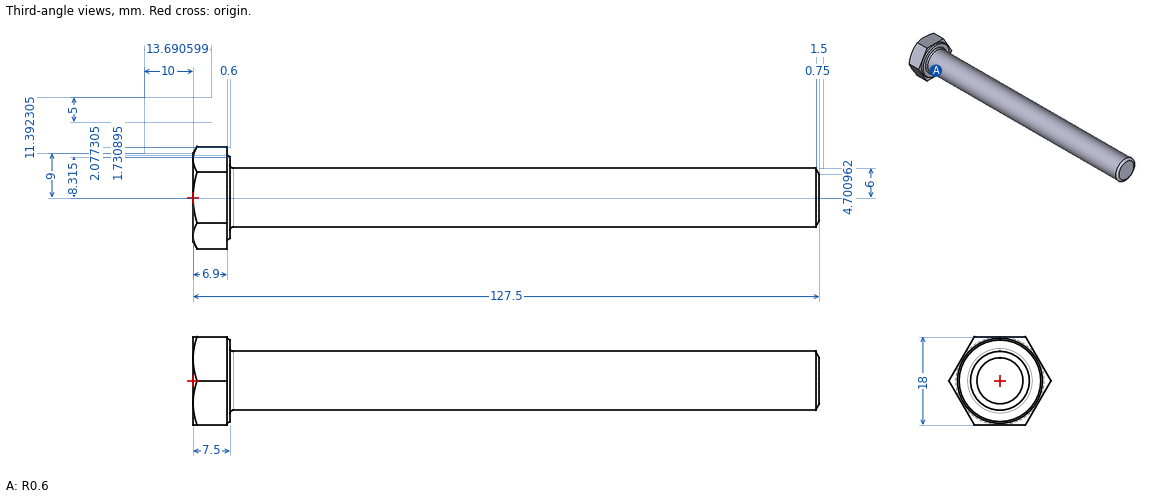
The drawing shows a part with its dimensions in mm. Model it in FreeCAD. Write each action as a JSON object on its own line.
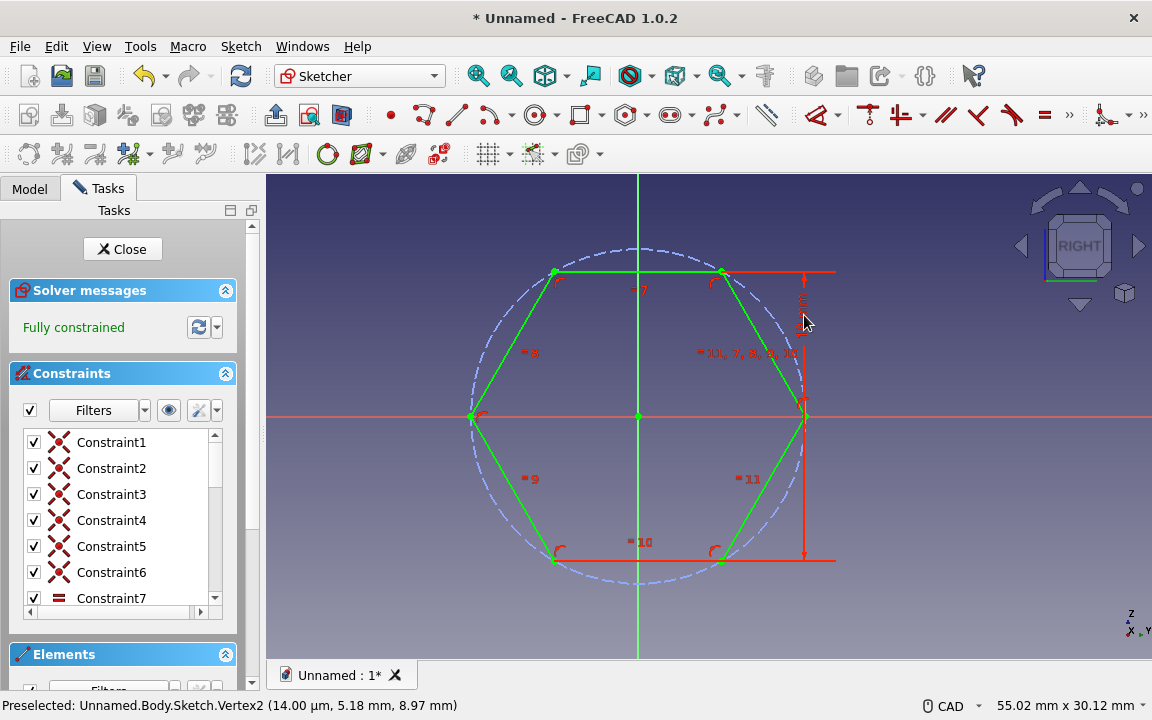
{"action": "left_click", "coordinate": [123, 249]}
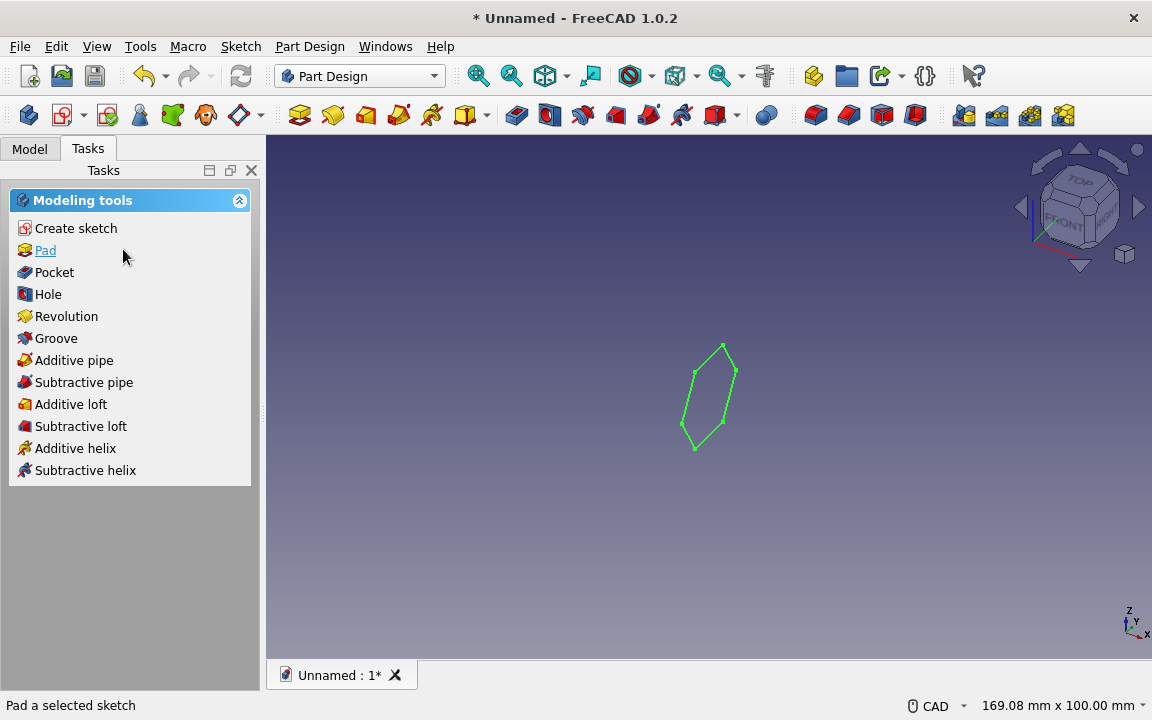
{"action": "left_click", "coordinate": [300, 116]}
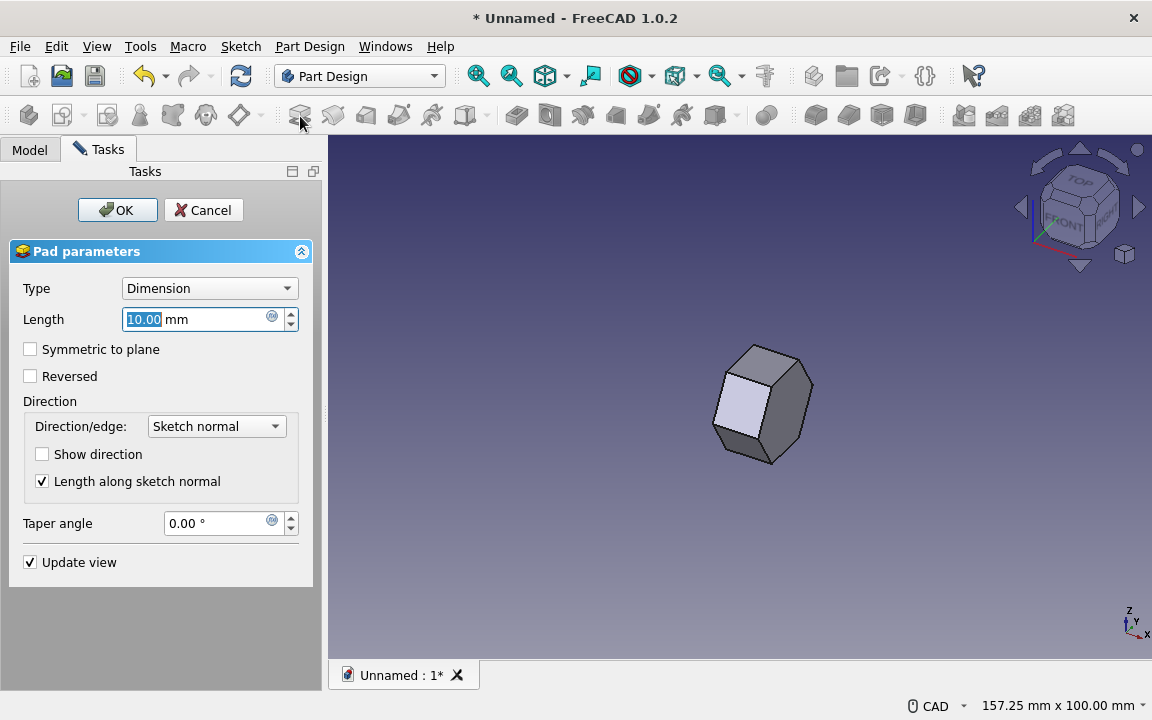
{"action": "type", "text": "7.5"}
{"action": "key", "text": "Tab"}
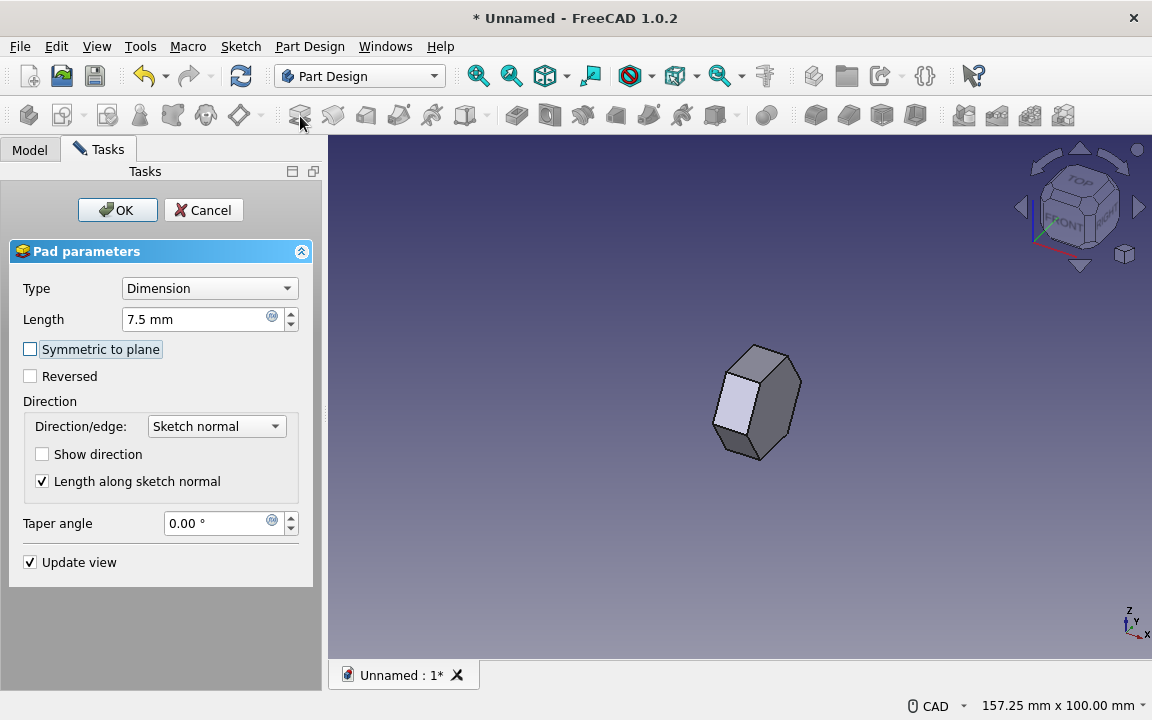
{"action": "left_click", "coordinate": [118, 210]}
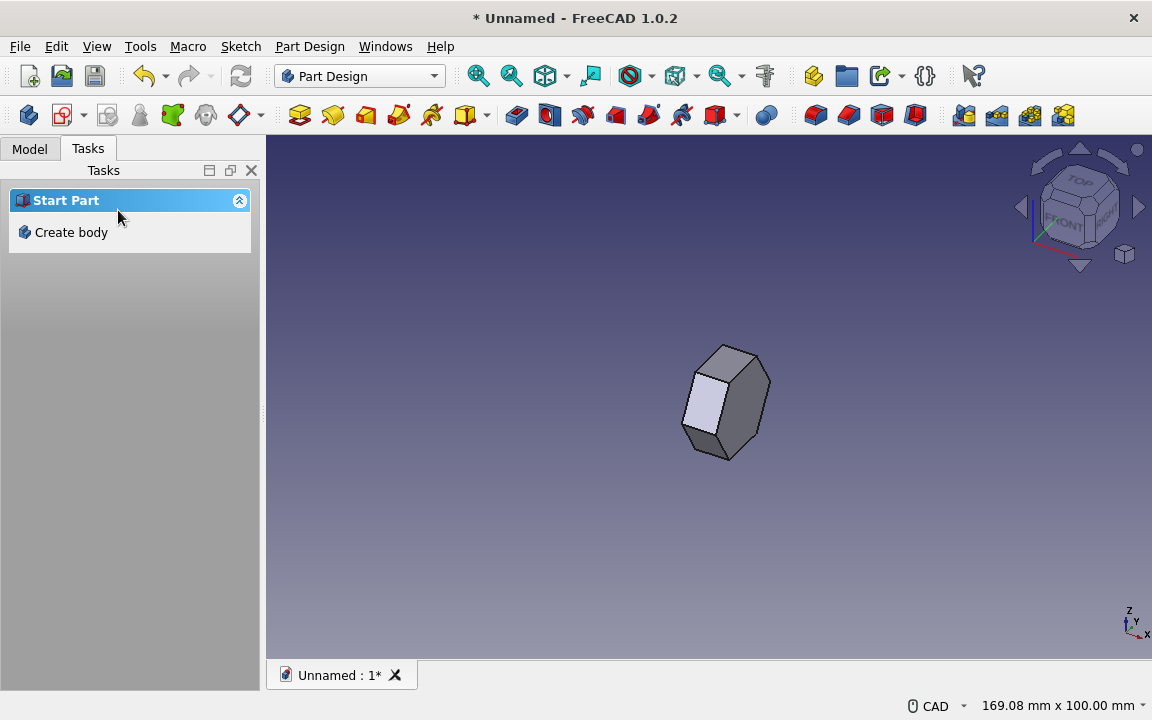
{"action": "left_click", "coordinate": [479, 76]}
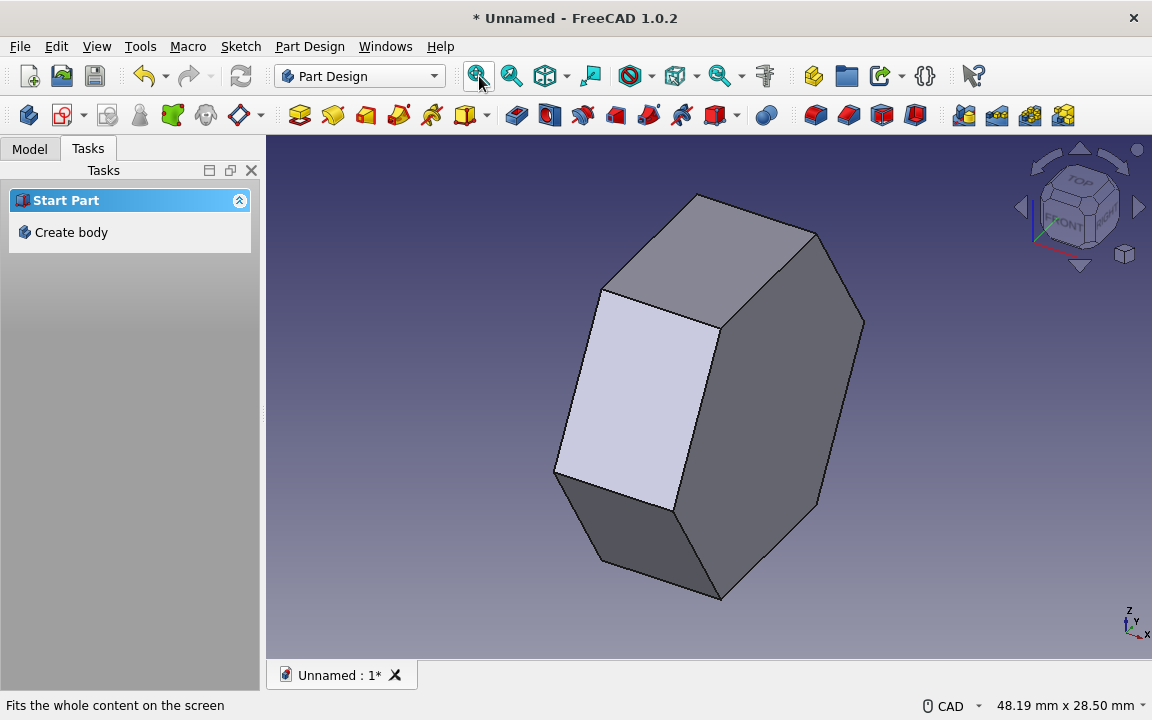
{"action": "left_click", "coordinate": [62, 116]}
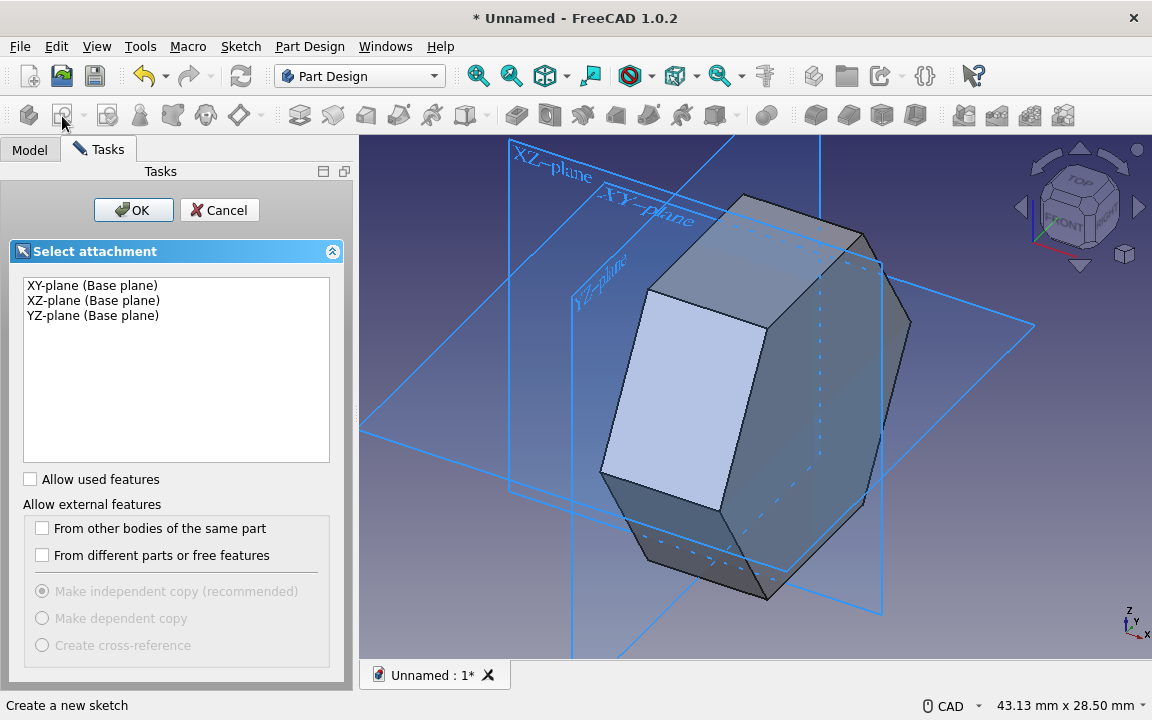
{"action": "left_click", "coordinate": [84, 286]}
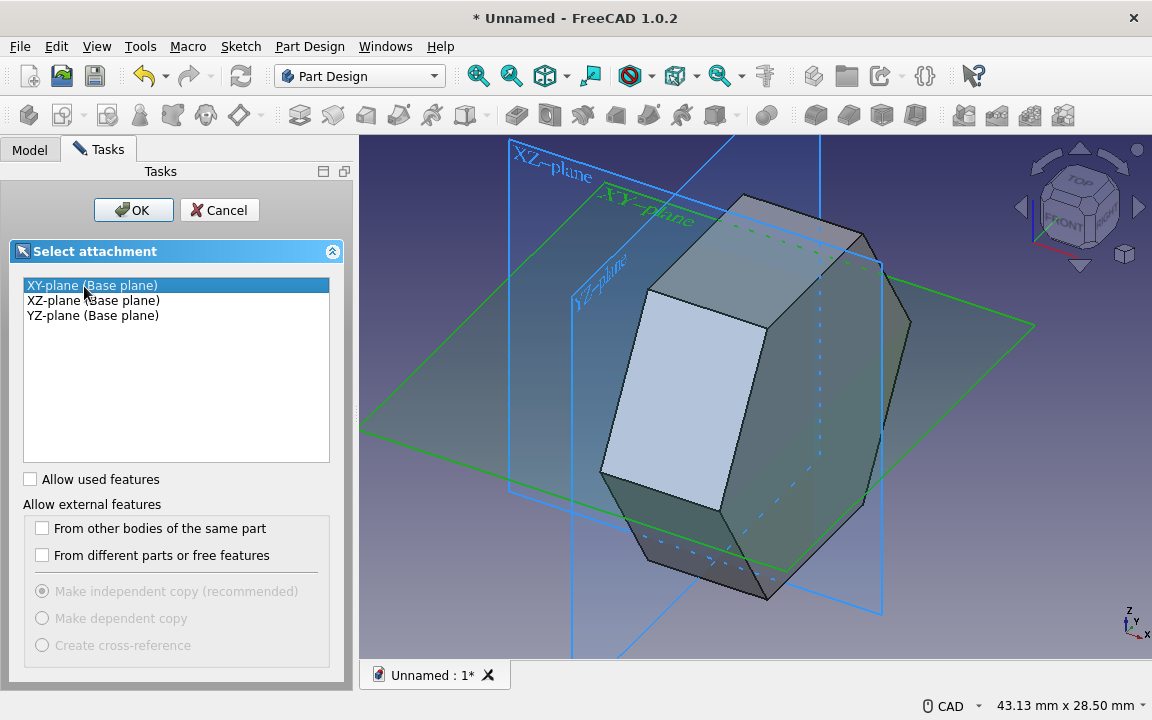
{"action": "left_click", "coordinate": [134, 210]}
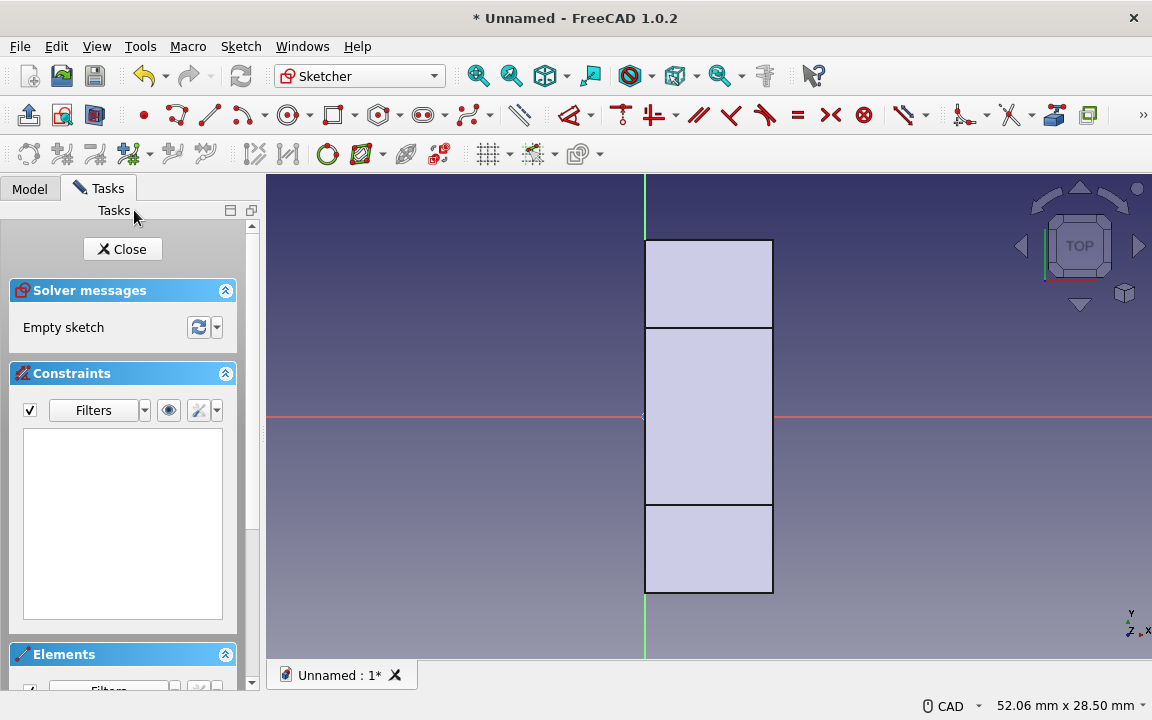
{"action": "left_click", "coordinate": [95, 116]}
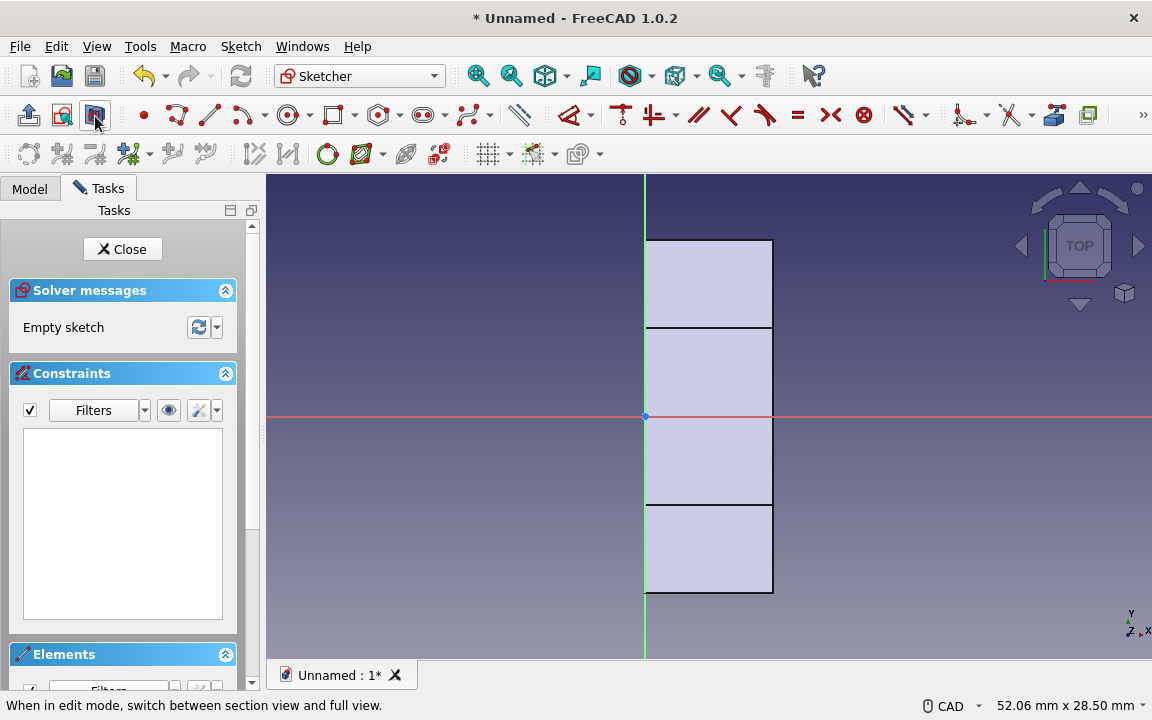
{"action": "scroll", "coordinate": [294, 433], "scroll_direction": "down", "scroll_amount": 7}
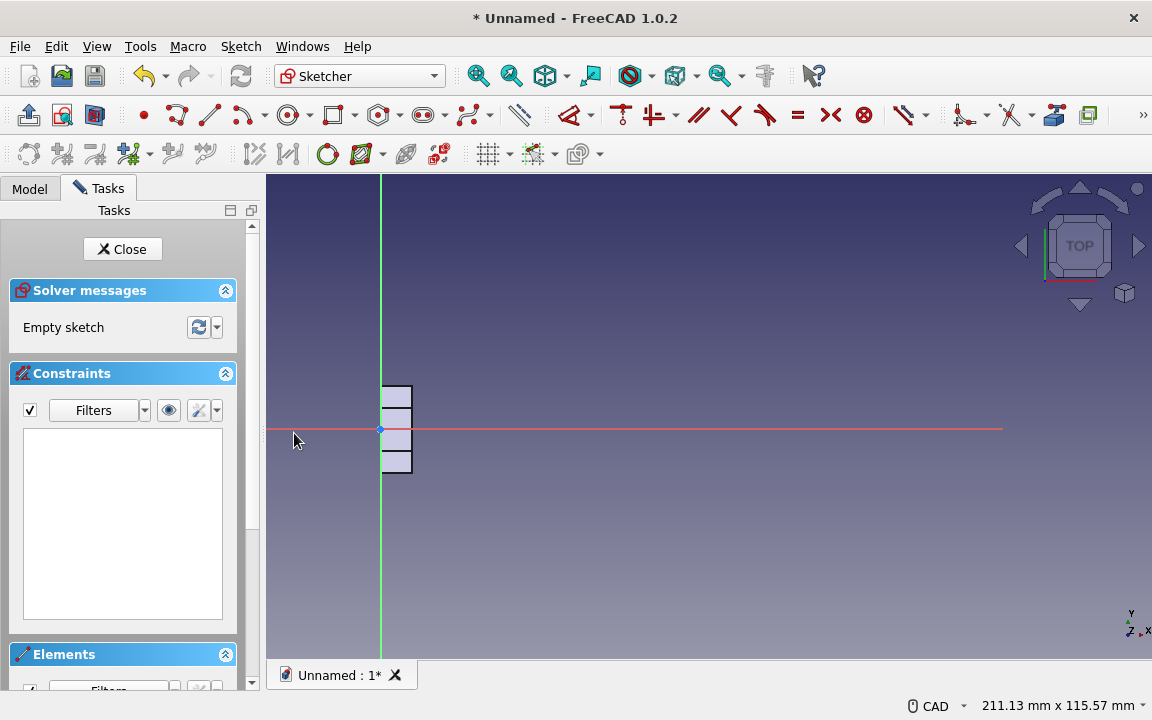
{"action": "left_click", "coordinate": [332, 116]}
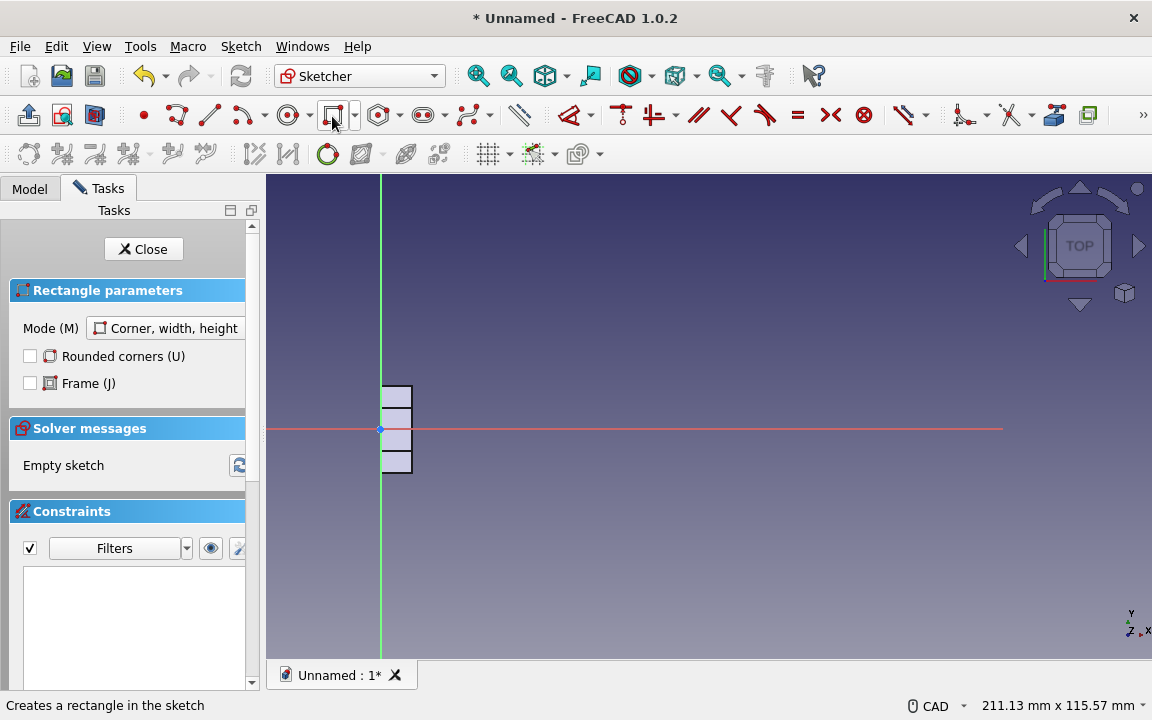
{"action": "left_click", "coordinate": [381, 429]}
{"action": "mouse_move", "coordinate": [916, 404]}